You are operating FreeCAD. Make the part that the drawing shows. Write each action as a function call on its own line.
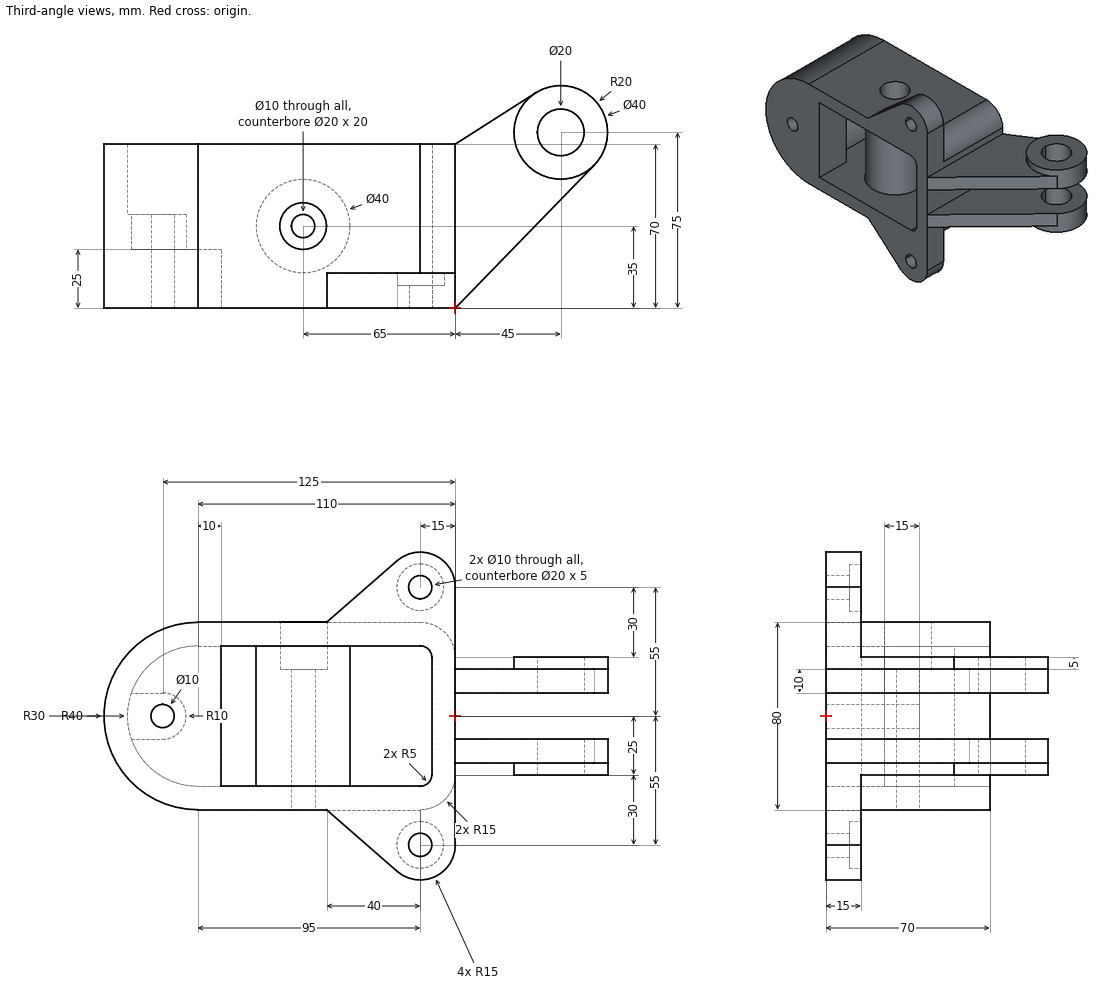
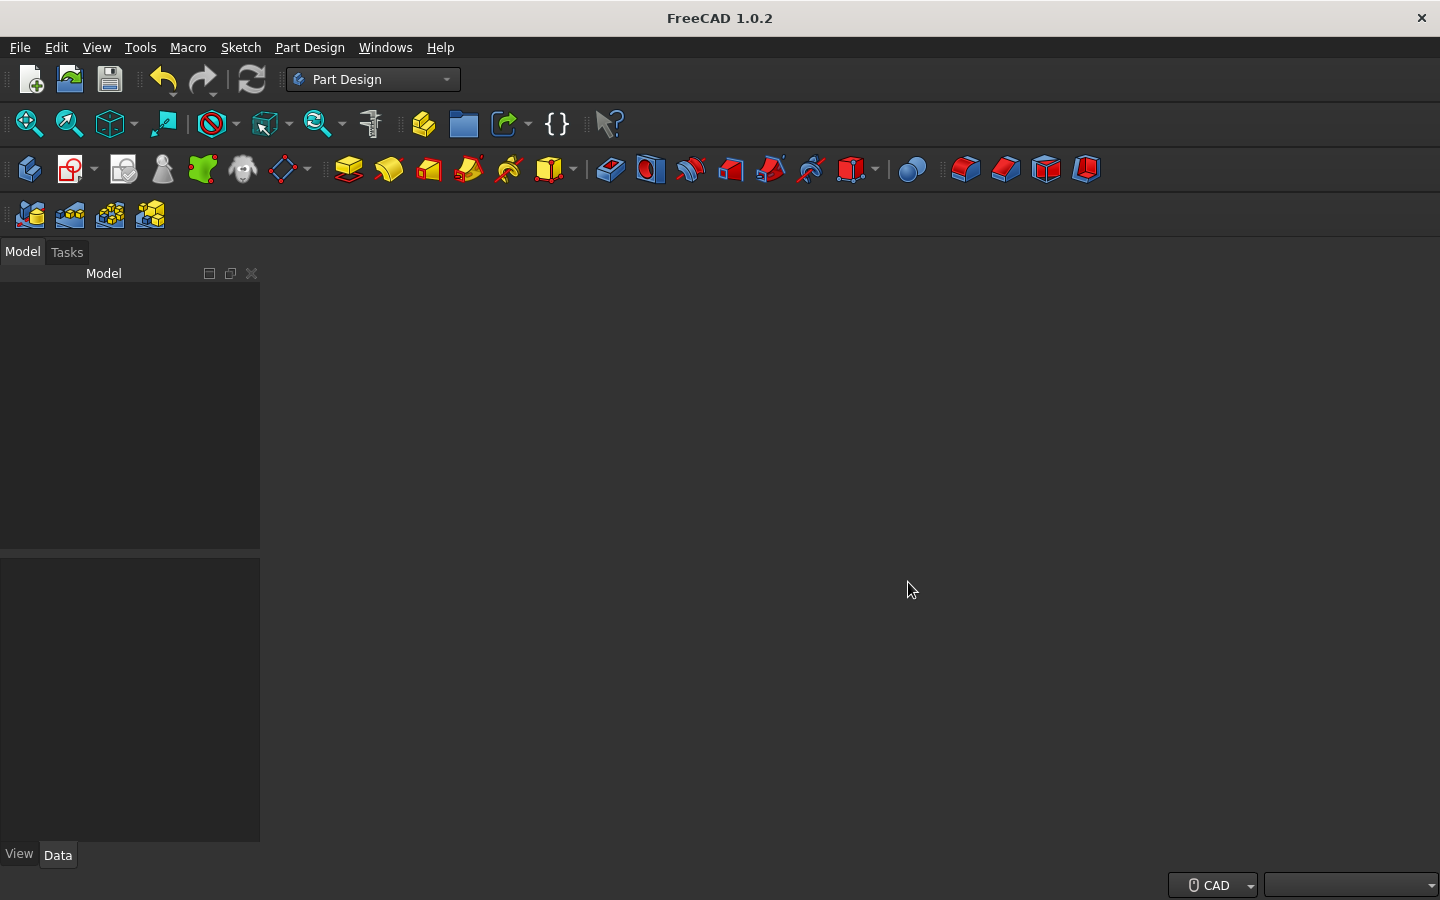
click(30, 80)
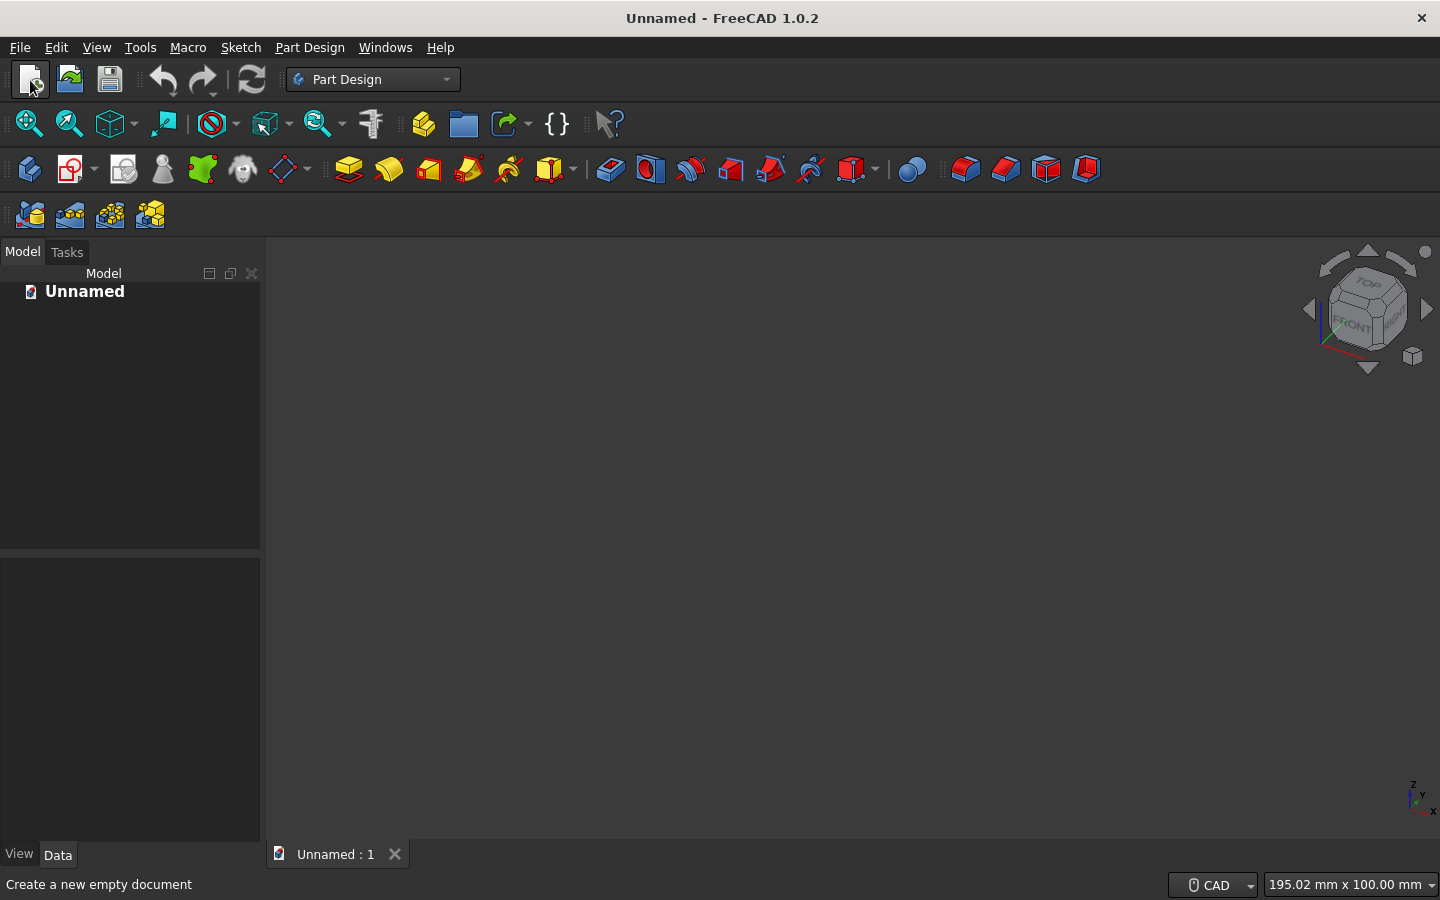
click(70, 170)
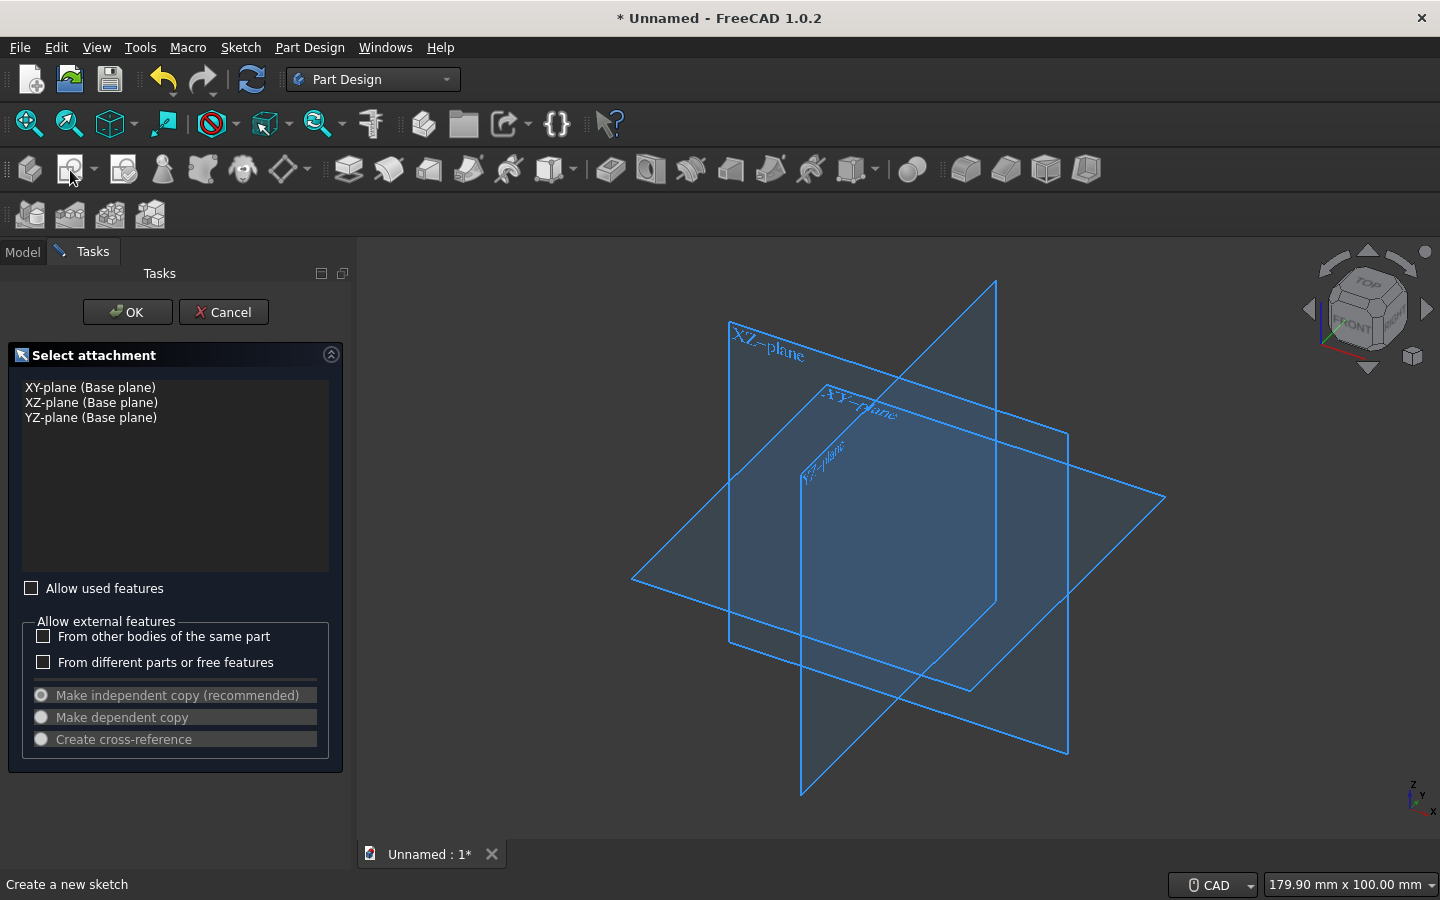
click(82, 402)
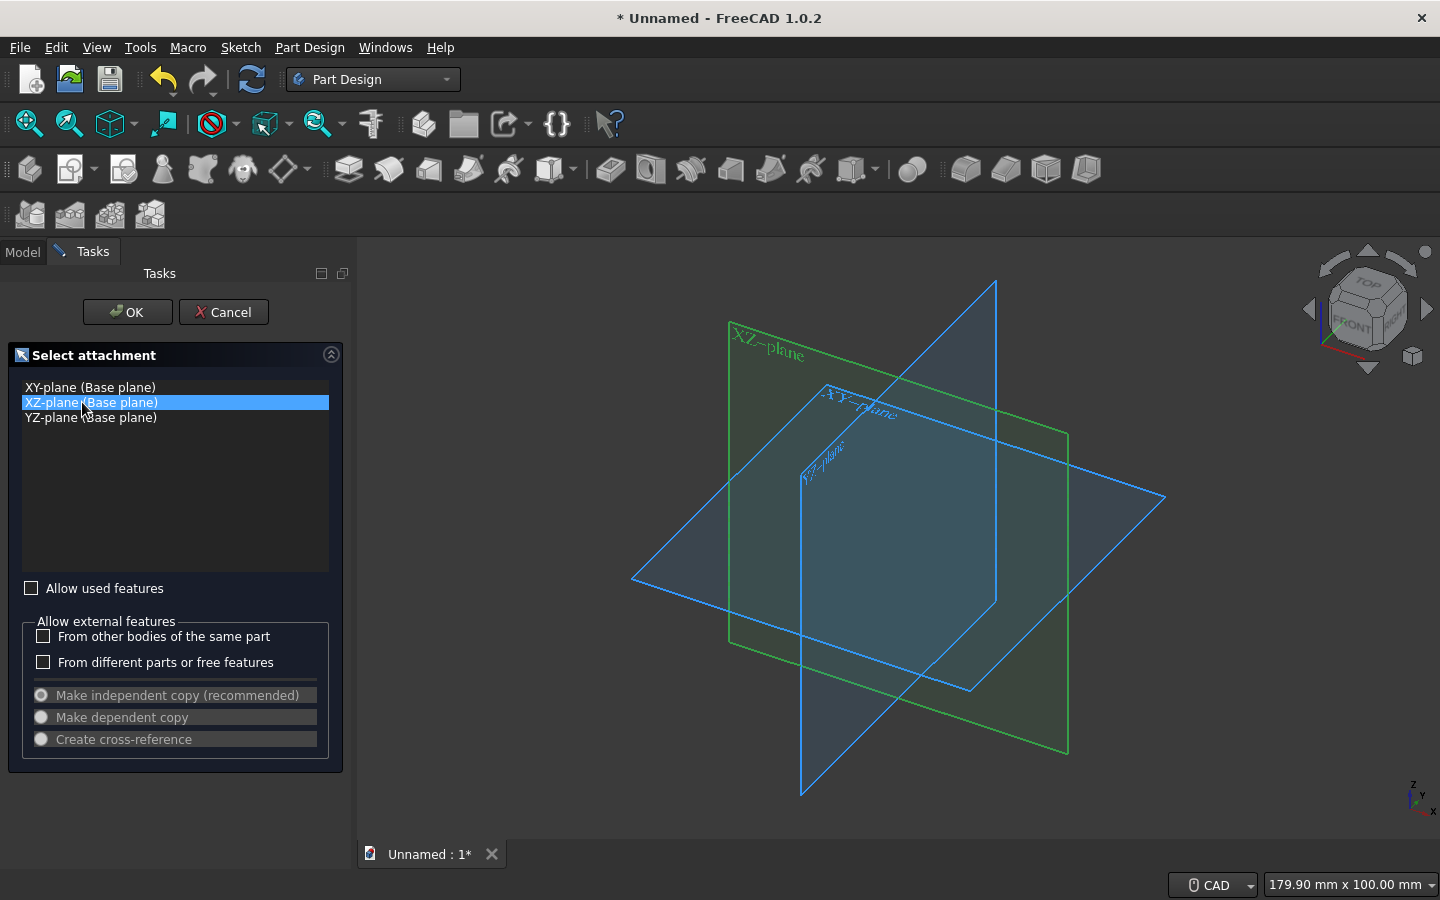
click(128, 312)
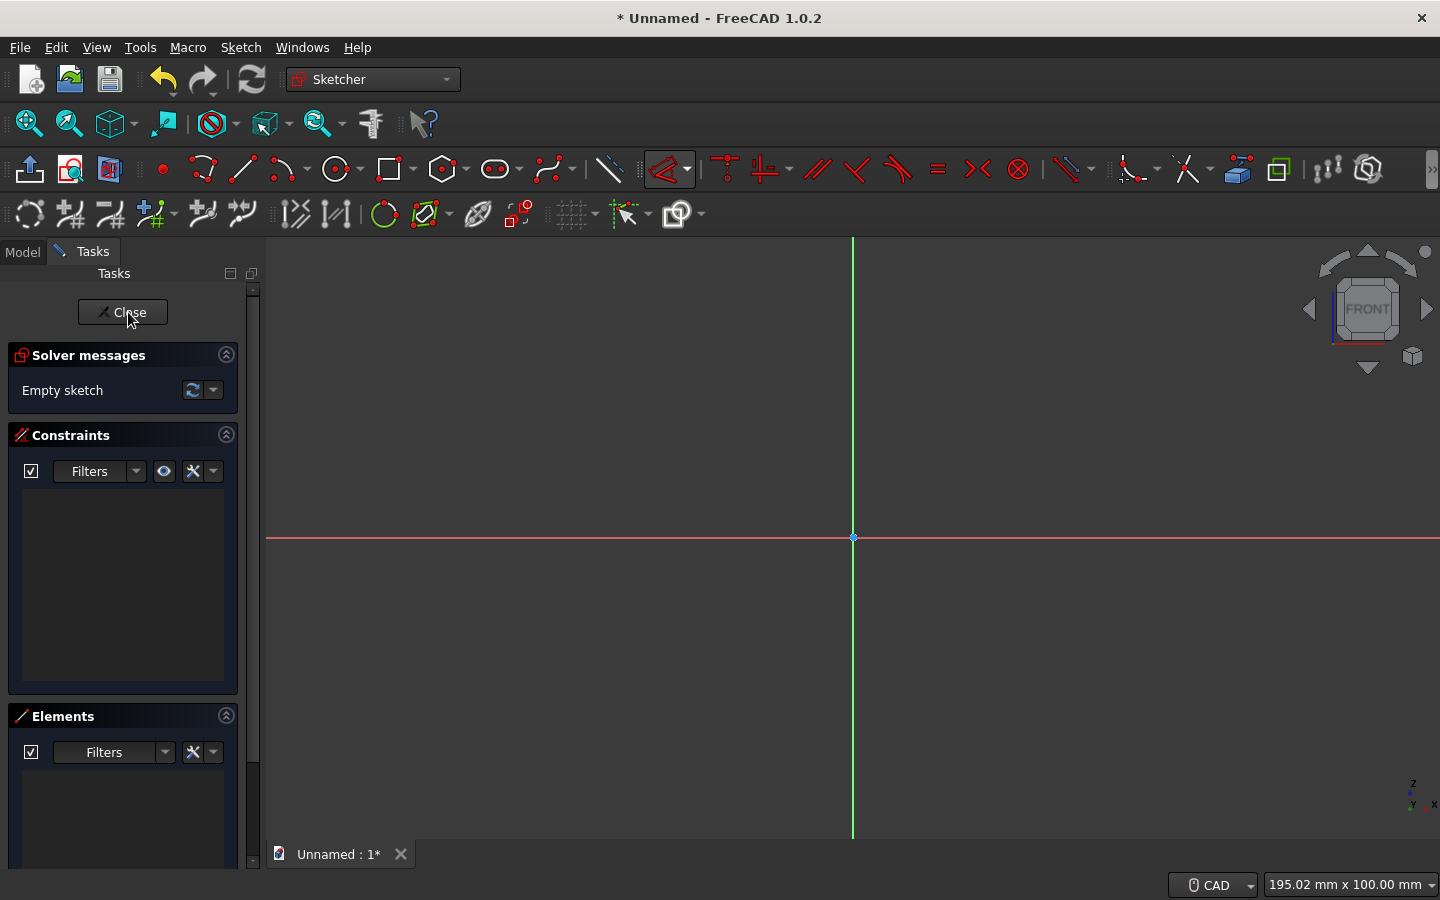
scroll(1275, 538, down, 2)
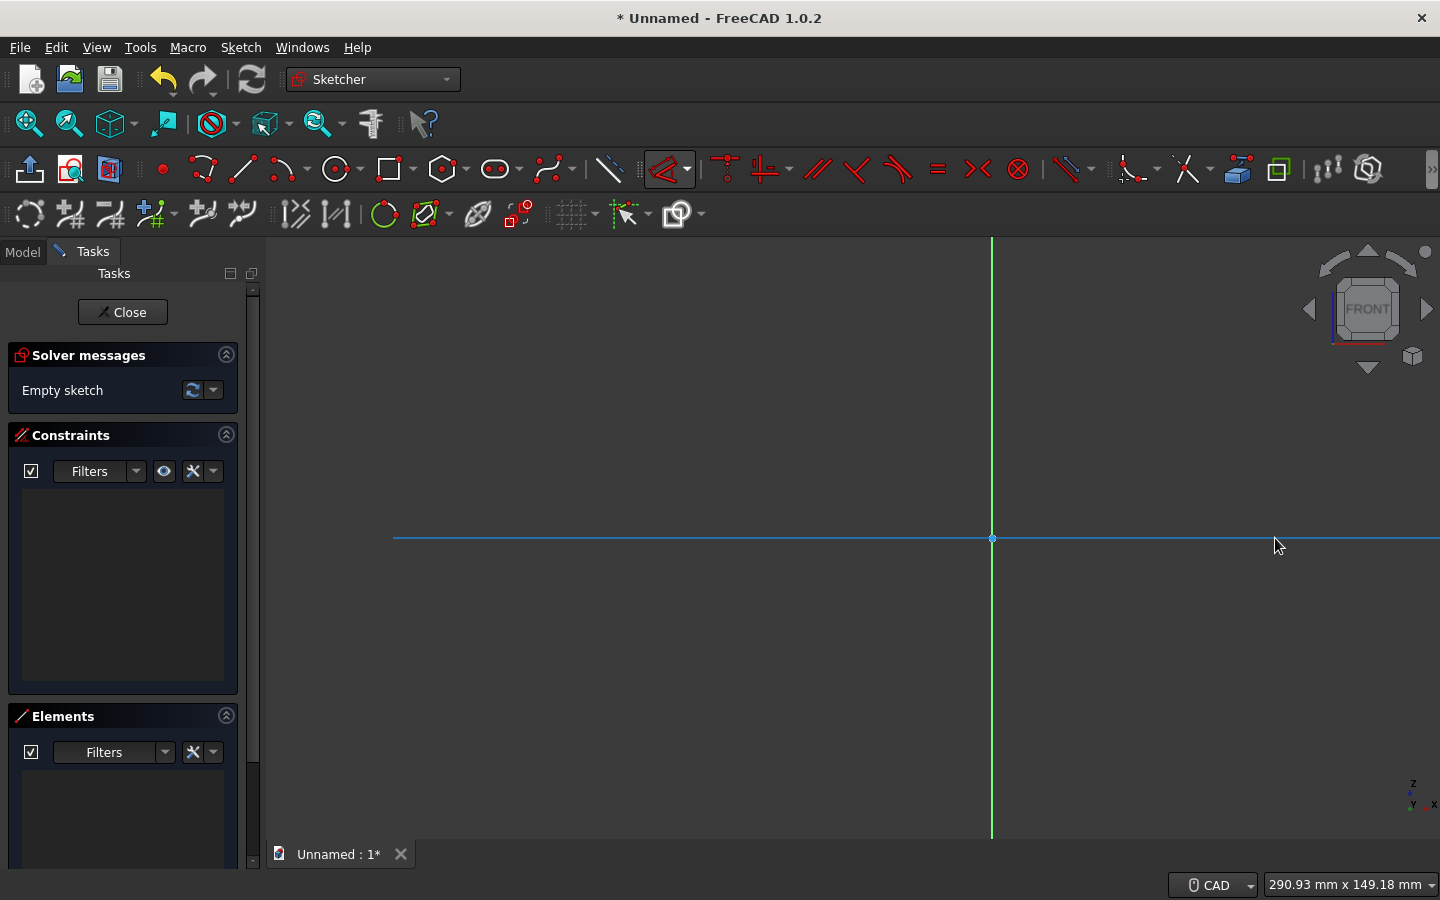
click(244, 170)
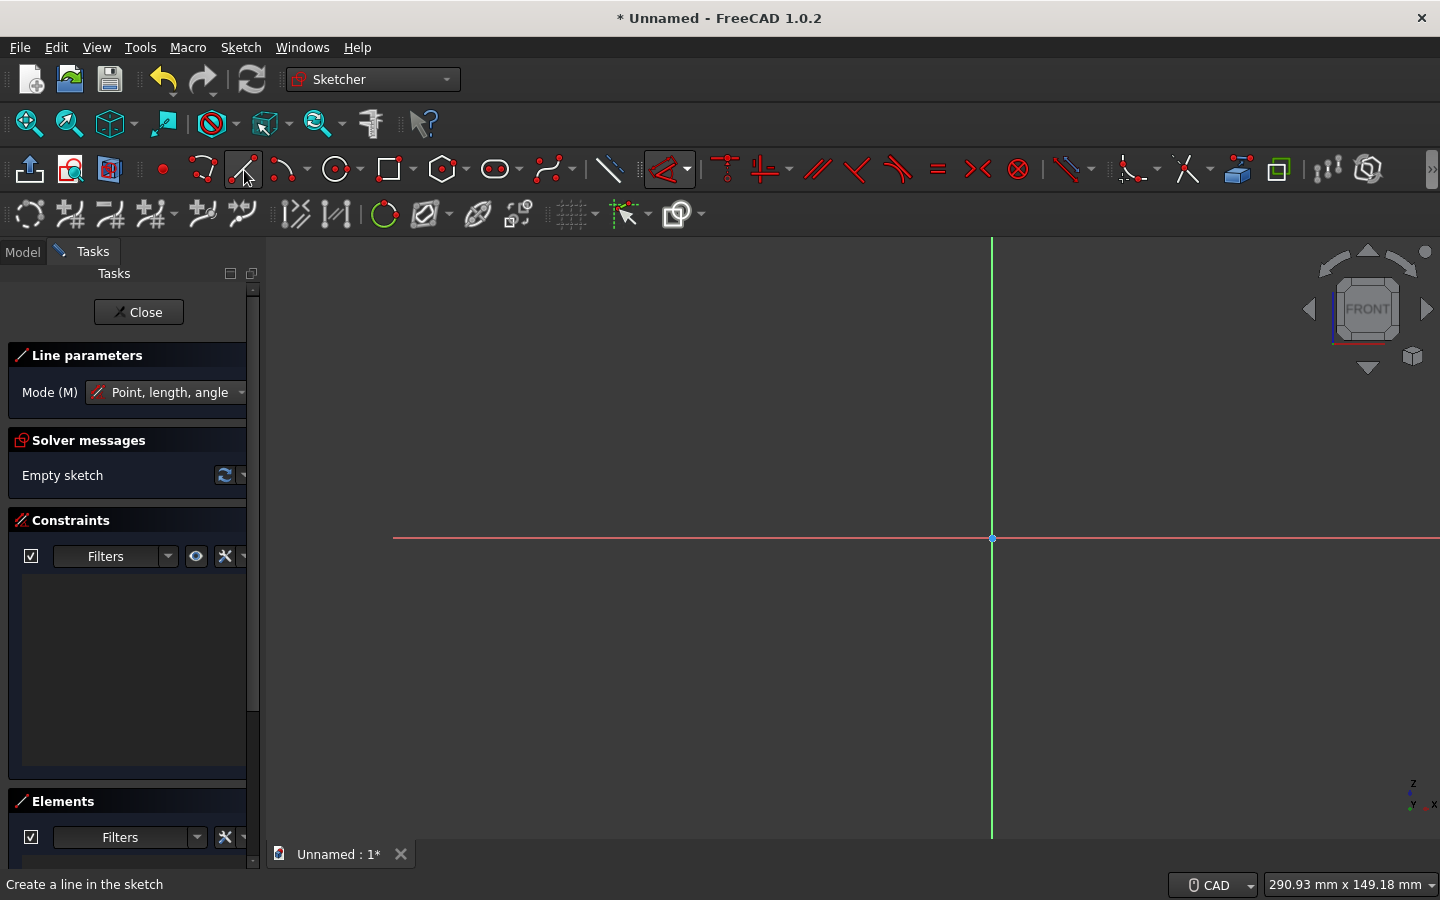
click(932, 700)
click(549, 700)